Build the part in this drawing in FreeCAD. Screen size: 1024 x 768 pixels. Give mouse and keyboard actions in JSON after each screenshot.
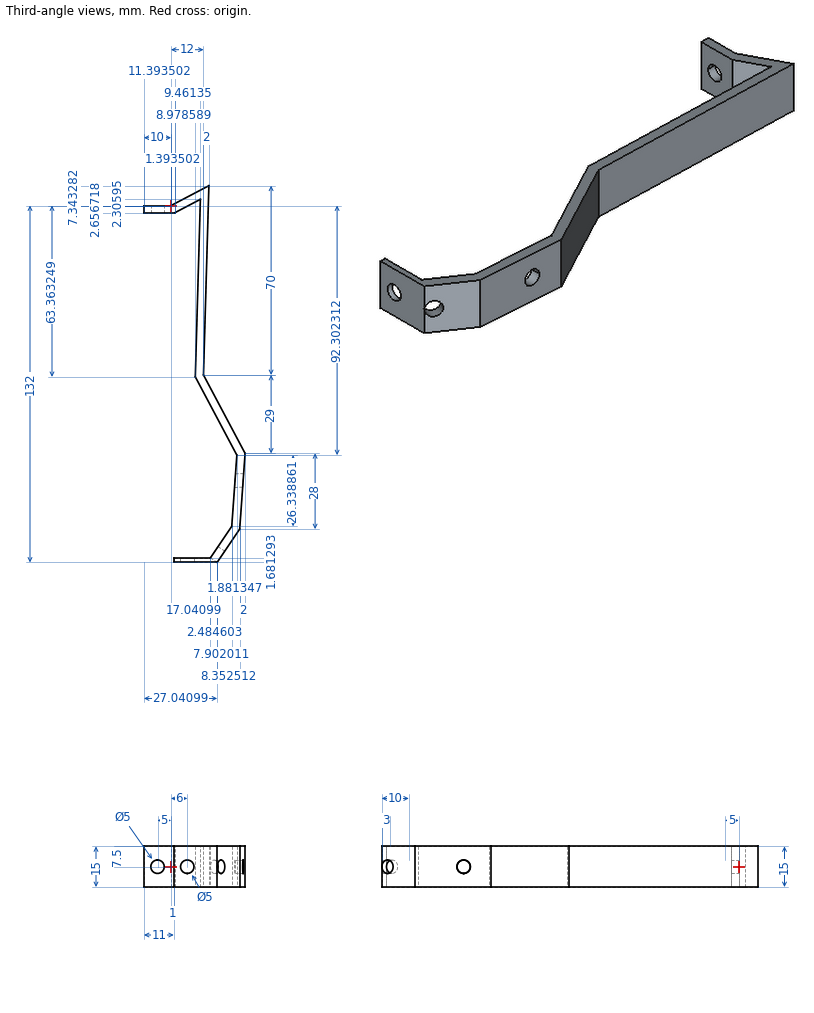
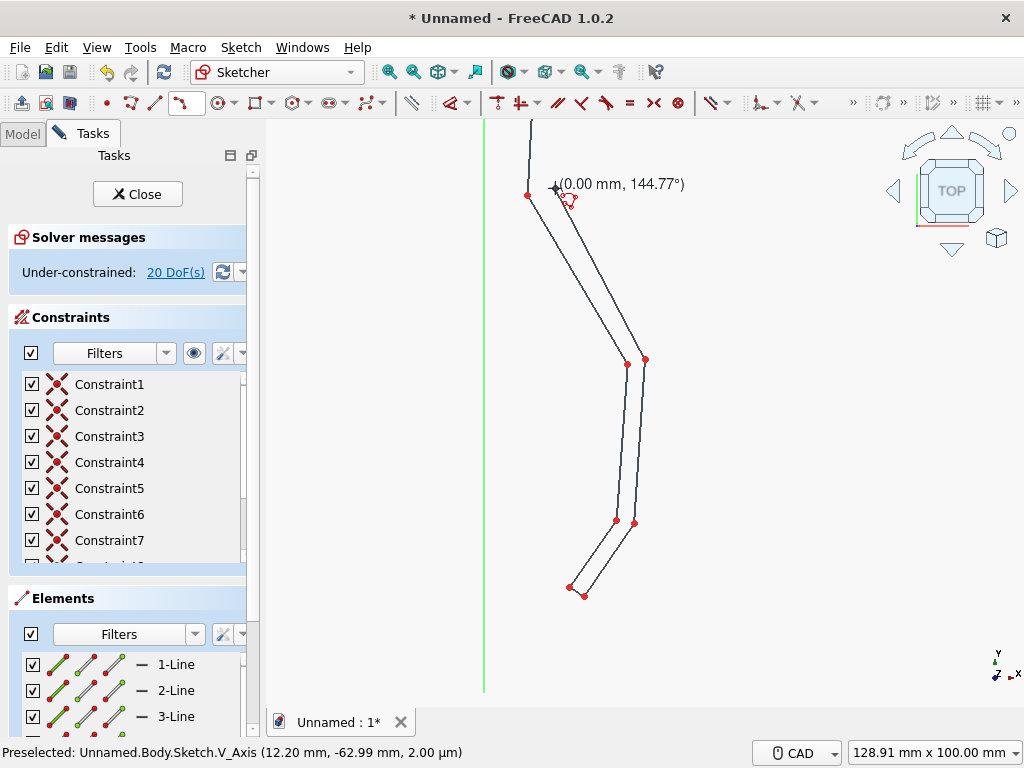
{"action": "scroll", "coordinate": [586, 598], "scroll_direction": "down", "scroll_amount": 4}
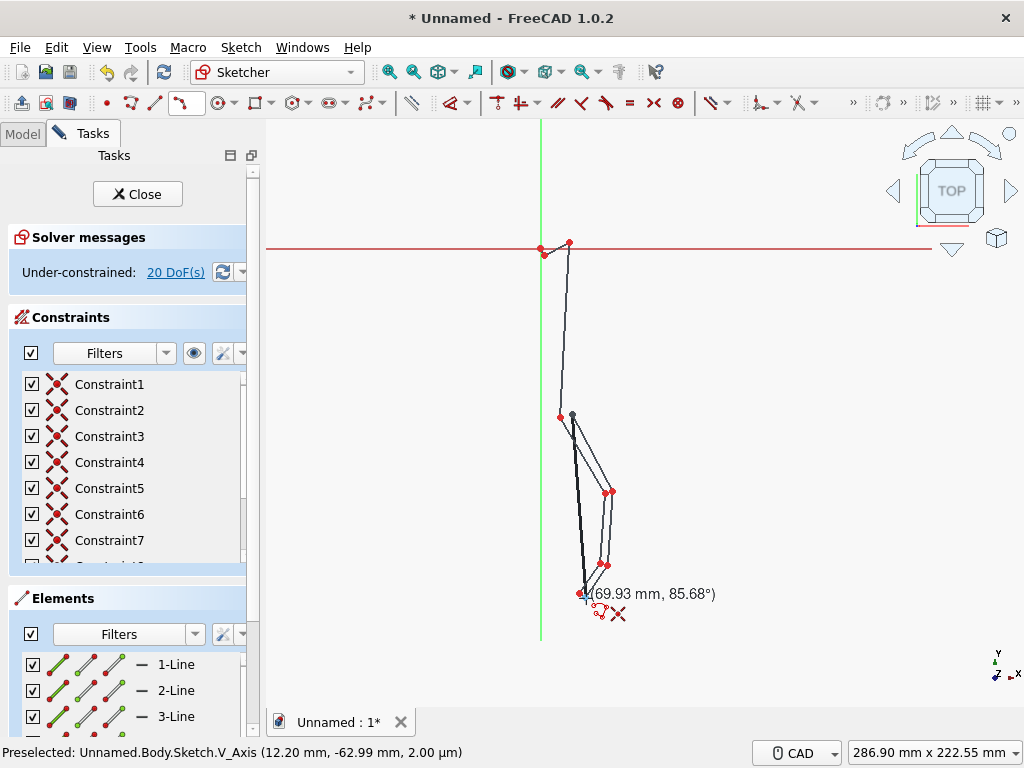
{"action": "left_click", "coordinate": [582, 229]}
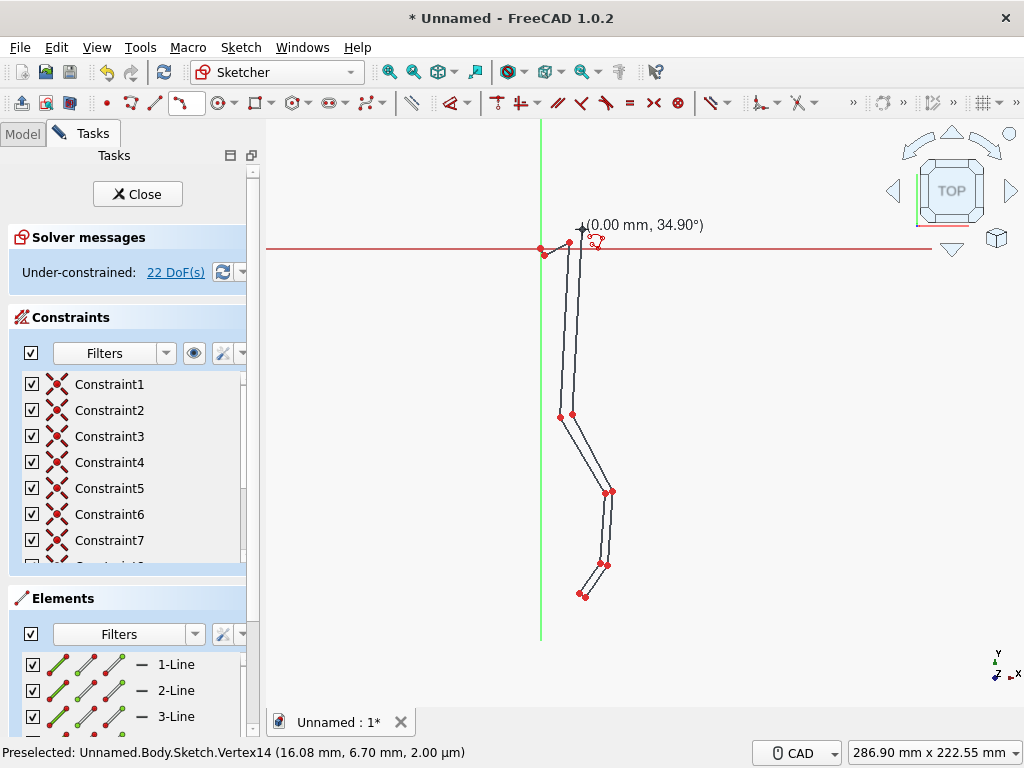
{"action": "scroll", "coordinate": [541, 249], "scroll_direction": "up", "scroll_amount": 7}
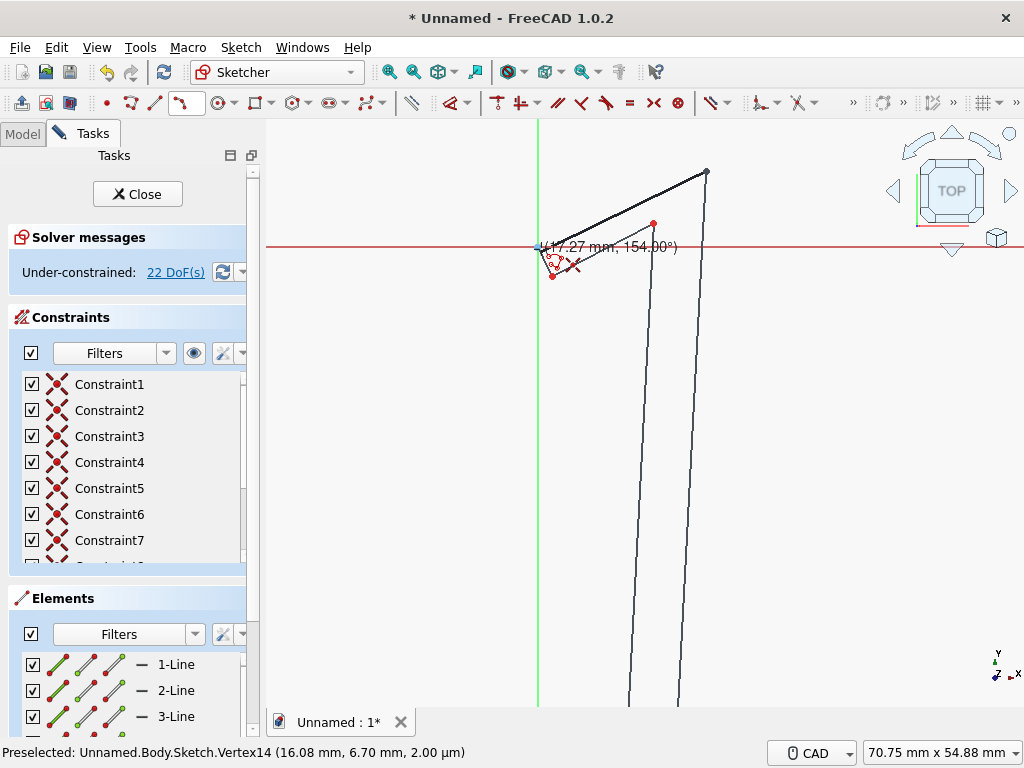
{"action": "left_click", "coordinate": [538, 247]}
{"action": "key", "text": "Escape"}
{"action": "key", "text": "Escape"}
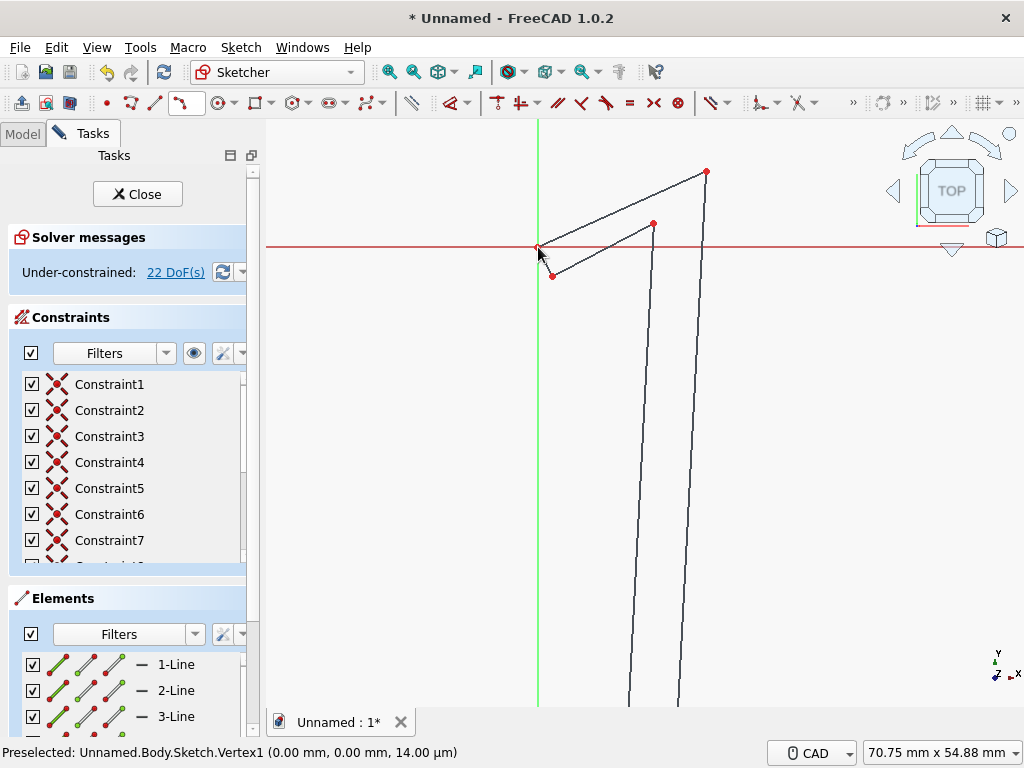
{"action": "left_click", "coordinate": [450, 104]}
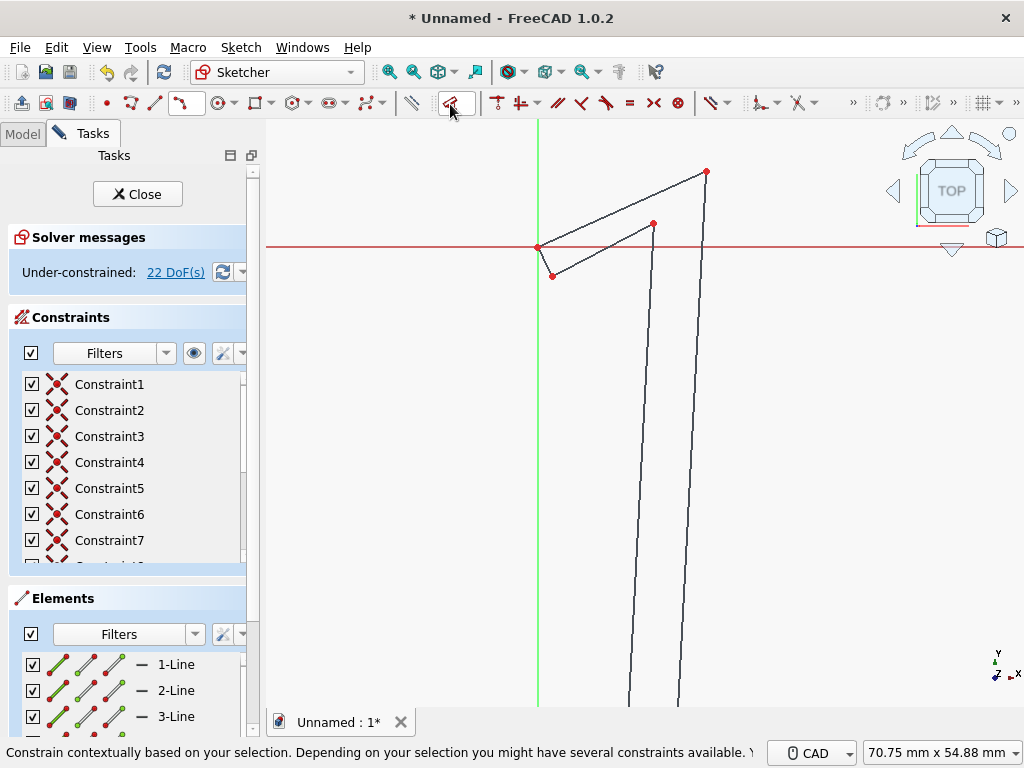
{"action": "scroll", "coordinate": [541, 249], "scroll_direction": "down", "scroll_amount": 7}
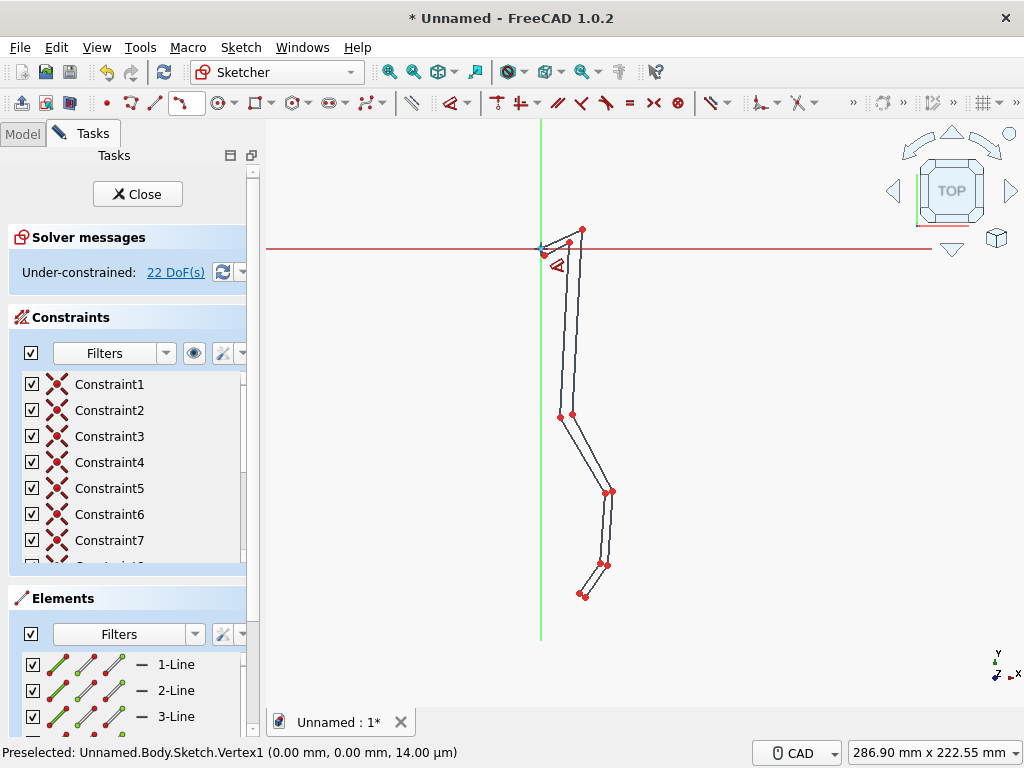
{"action": "scroll", "coordinate": [609, 543], "scroll_direction": "up", "scroll_amount": 11}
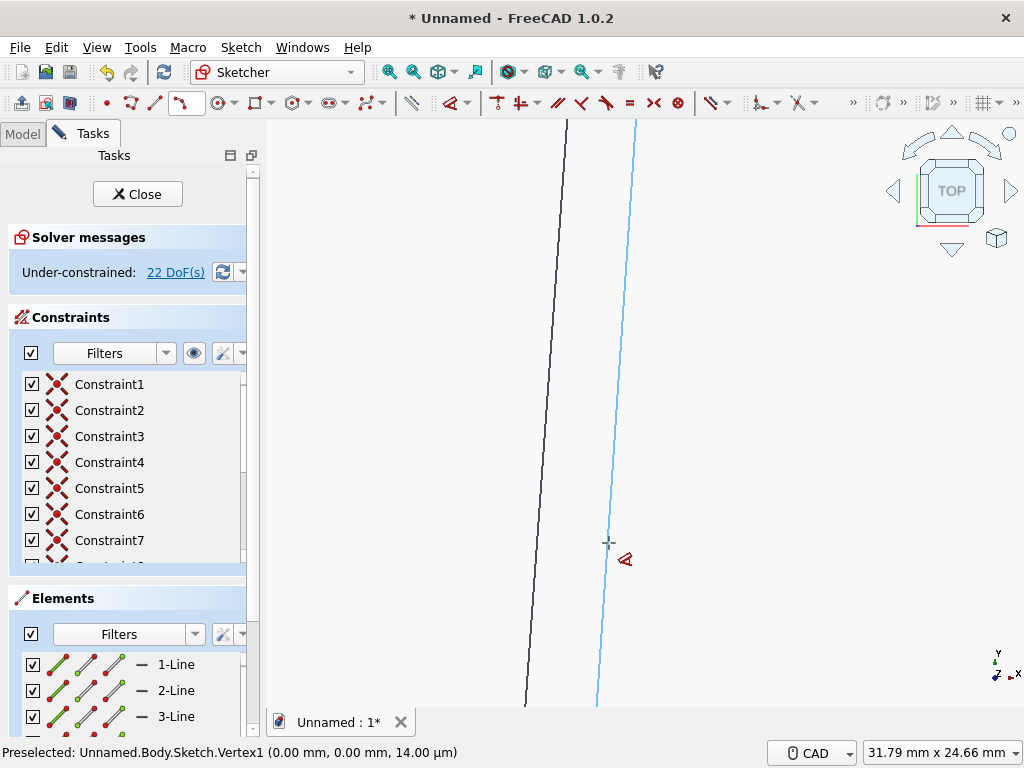
{"action": "left_click", "coordinate": [608, 538]}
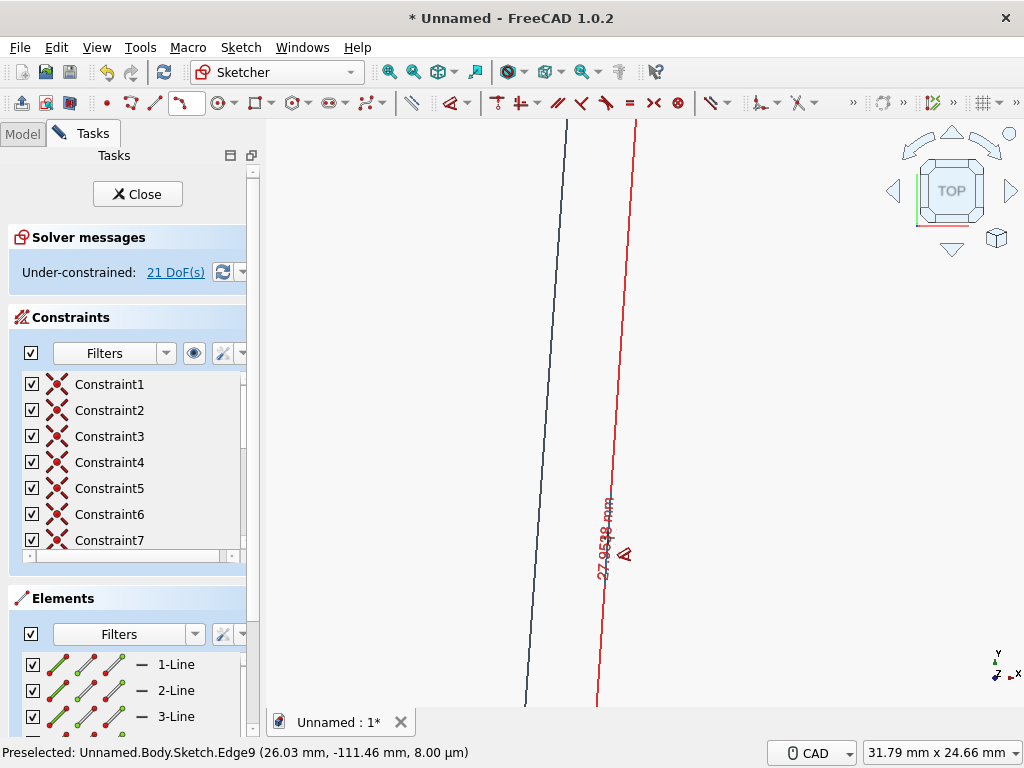
{"action": "key", "text": "Escape"}
{"action": "key", "text": "Escape"}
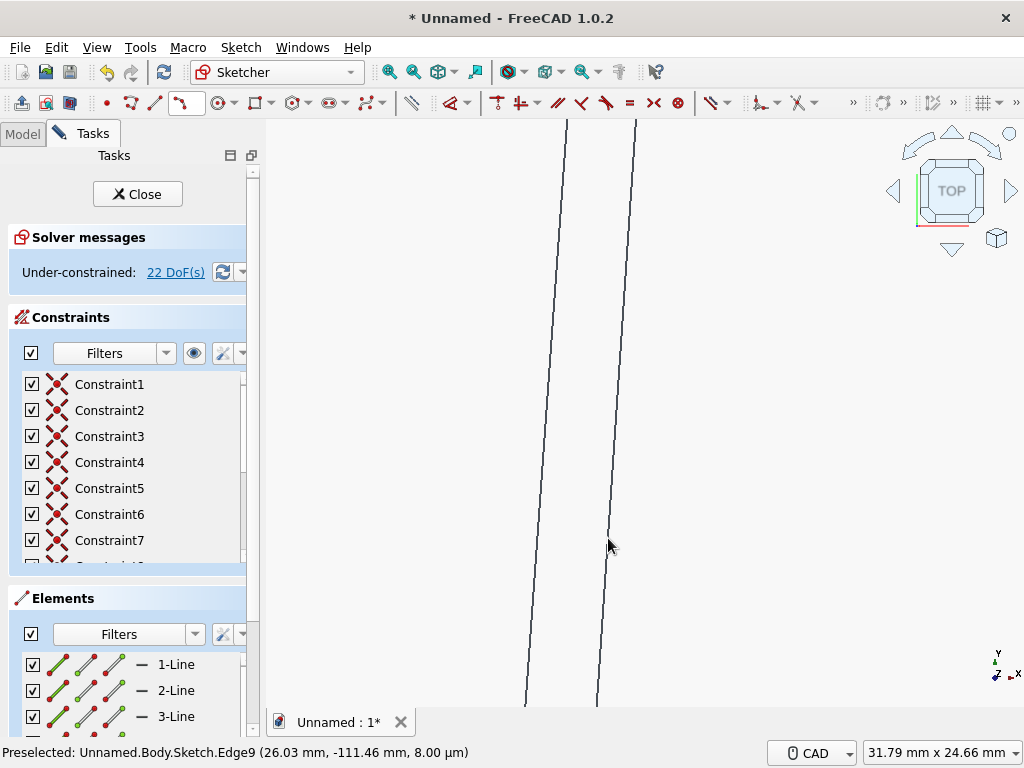
{"action": "left_click", "coordinate": [608, 538]}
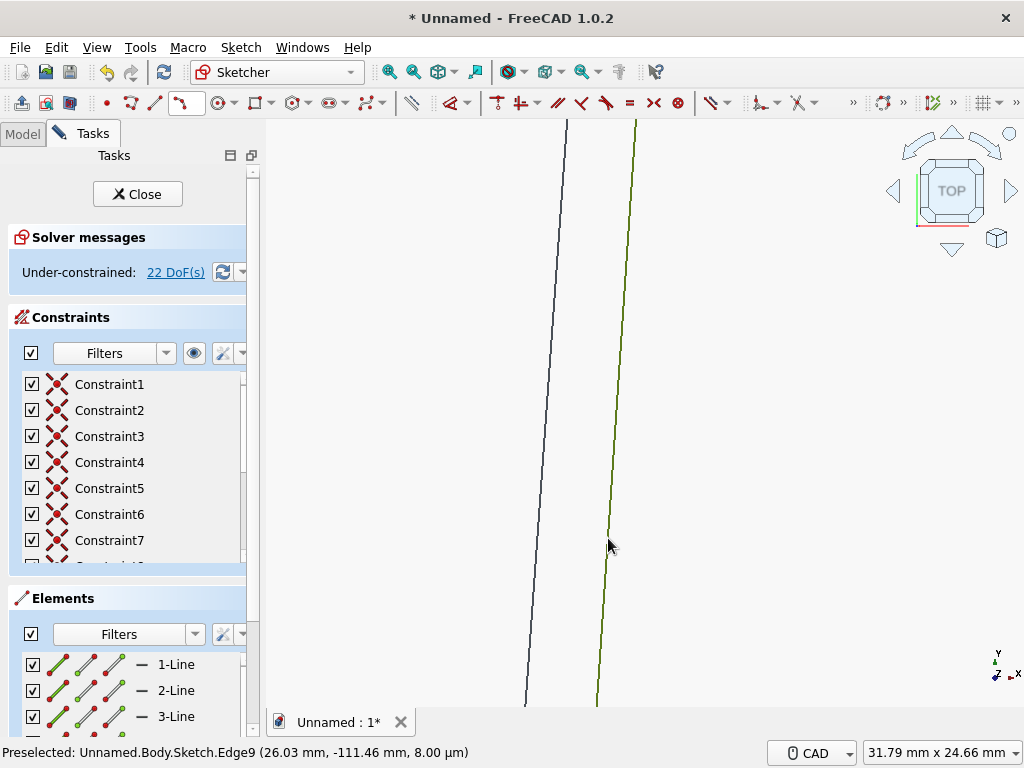
{"action": "left_click", "coordinate": [470, 104]}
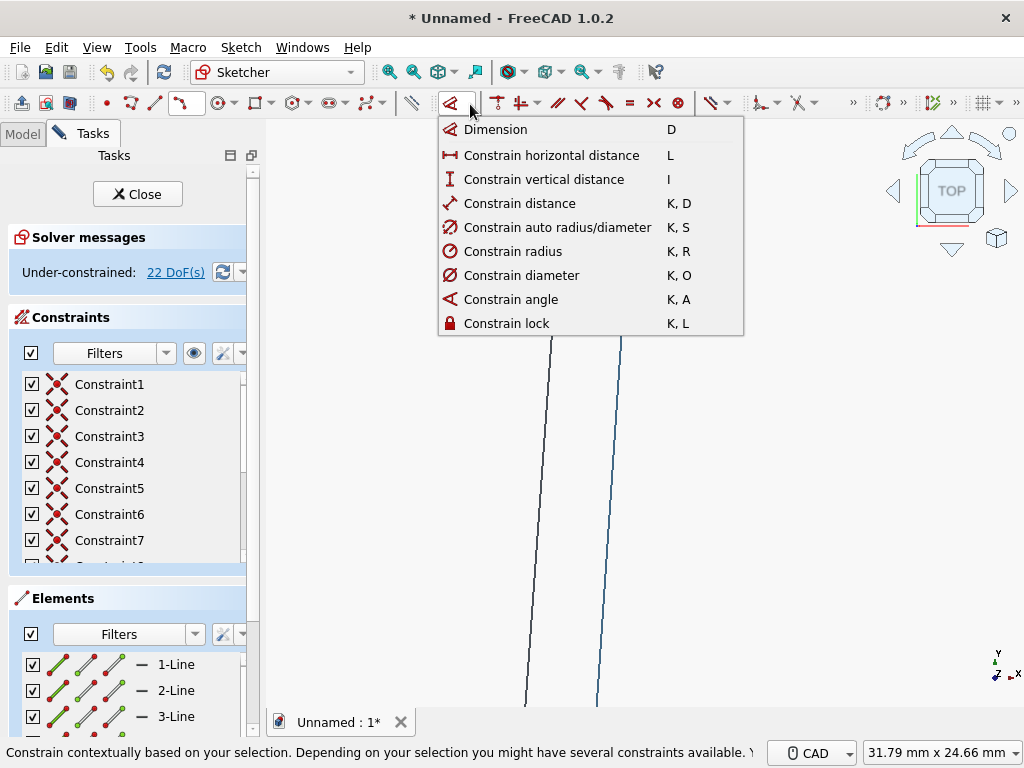
{"action": "left_click", "coordinate": [591, 155]}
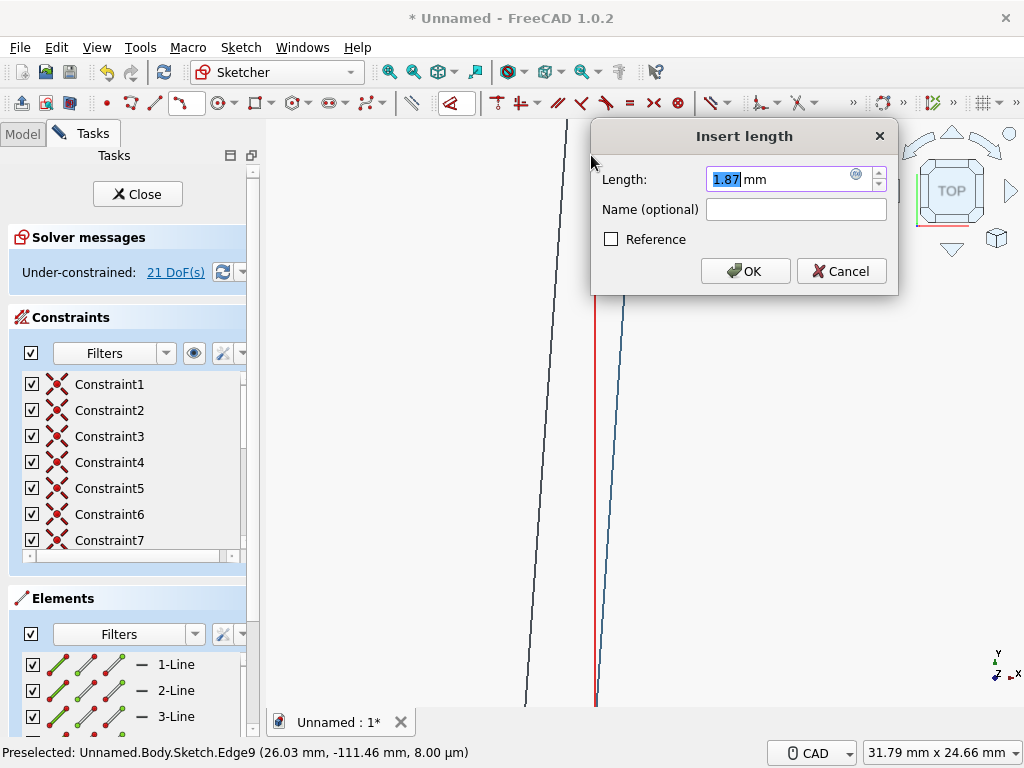
{"action": "type", "text": "2"}
{"action": "key", "text": "Return"}